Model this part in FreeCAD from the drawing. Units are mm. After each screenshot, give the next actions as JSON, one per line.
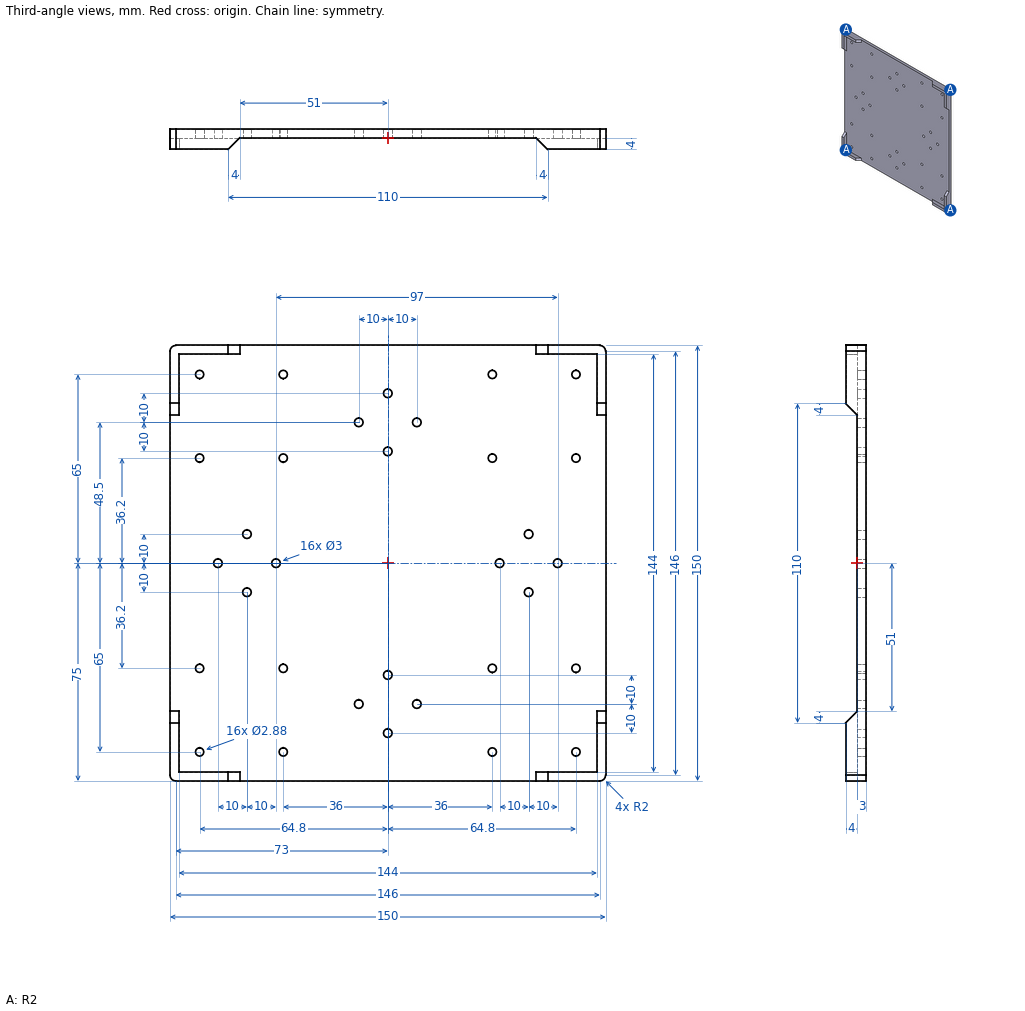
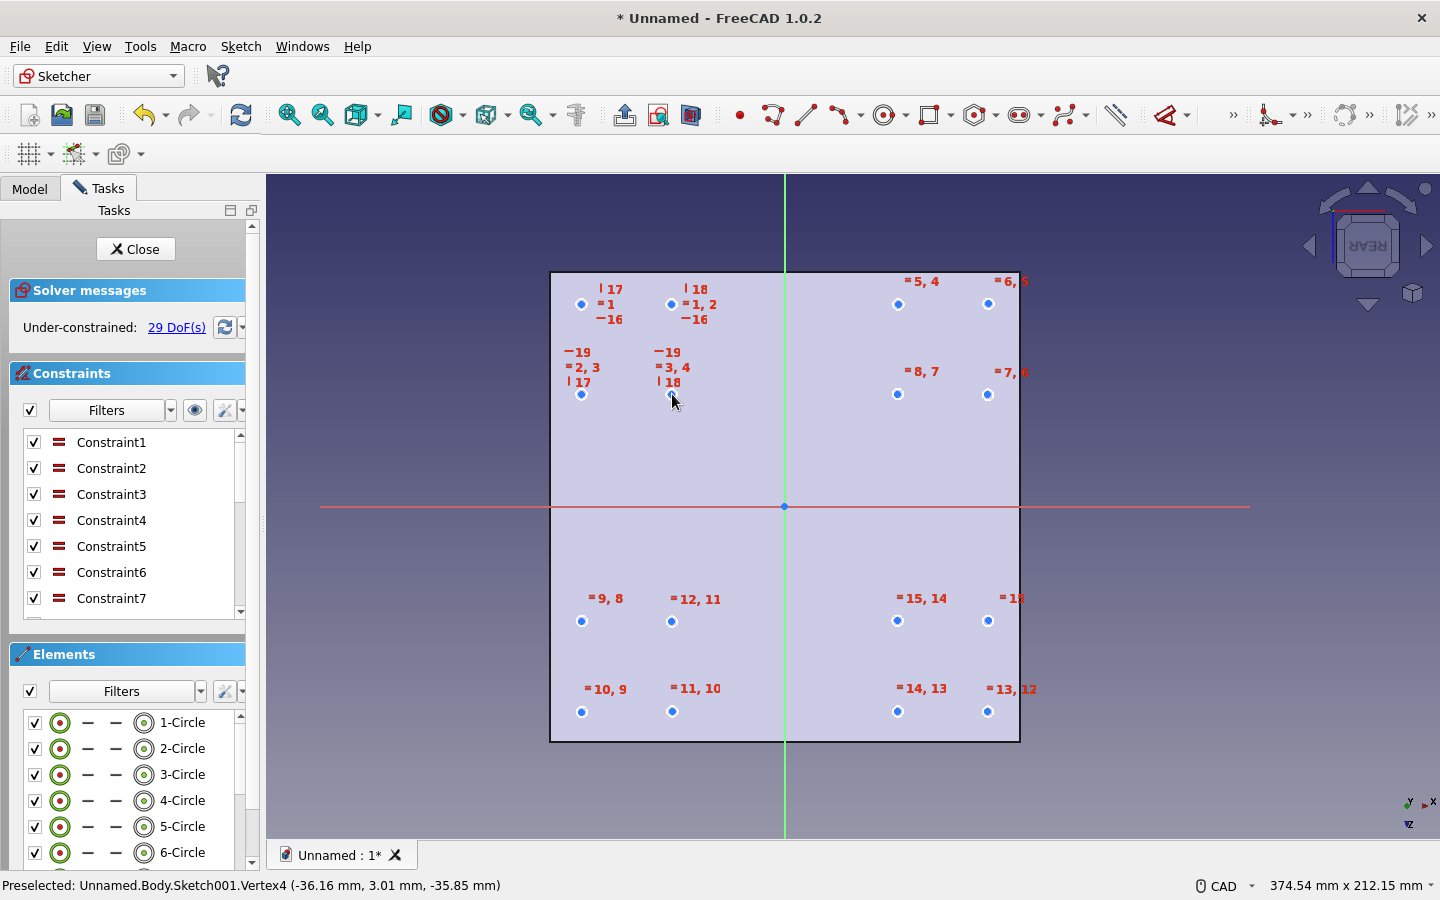
{"action": "left_click", "coordinate": [672, 304]}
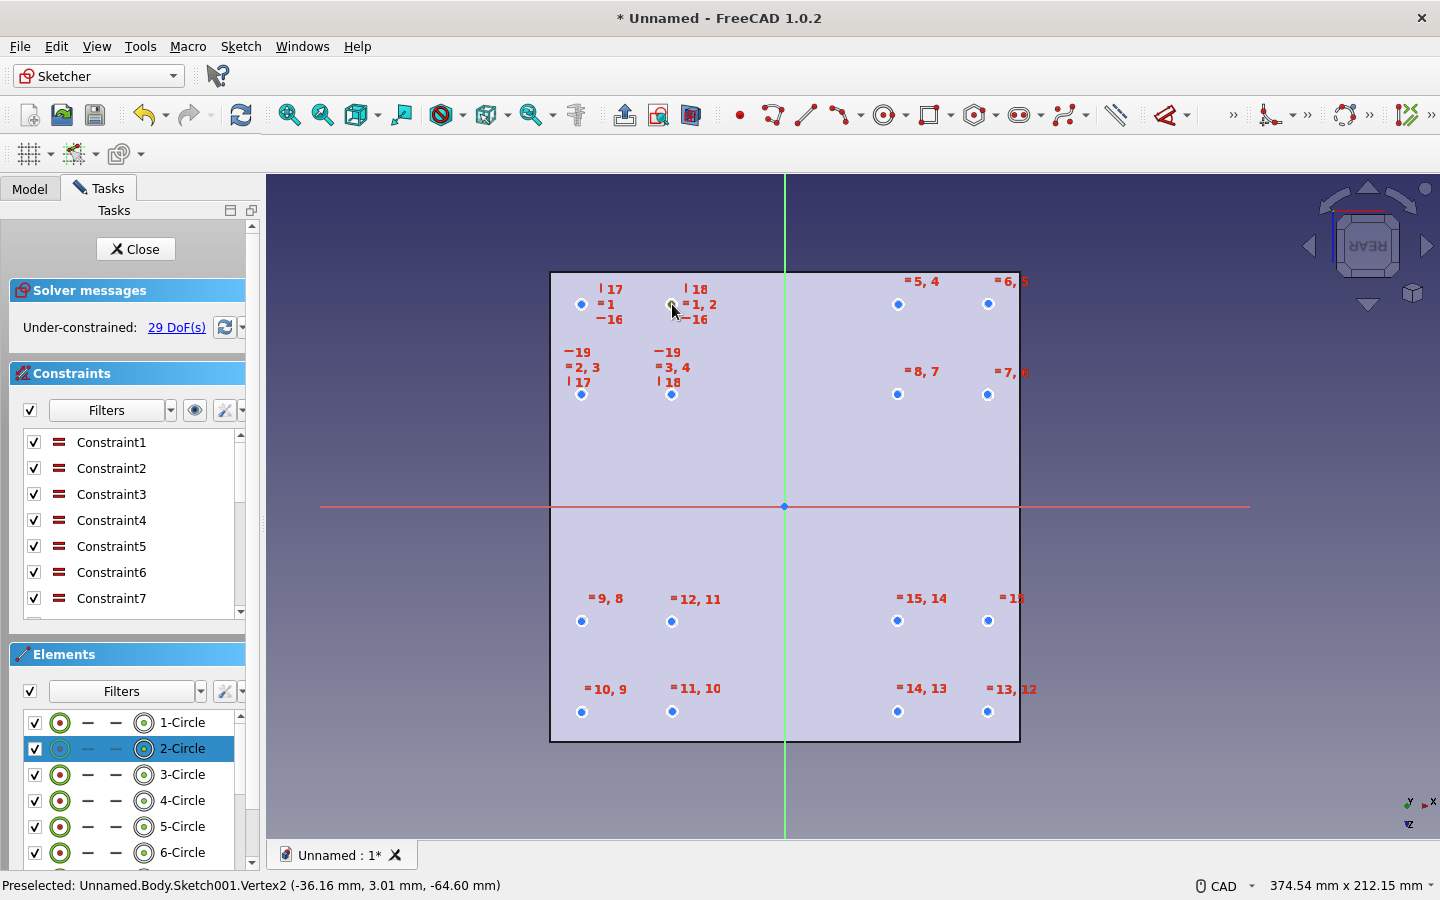
{"action": "left_click", "coordinate": [898, 304]}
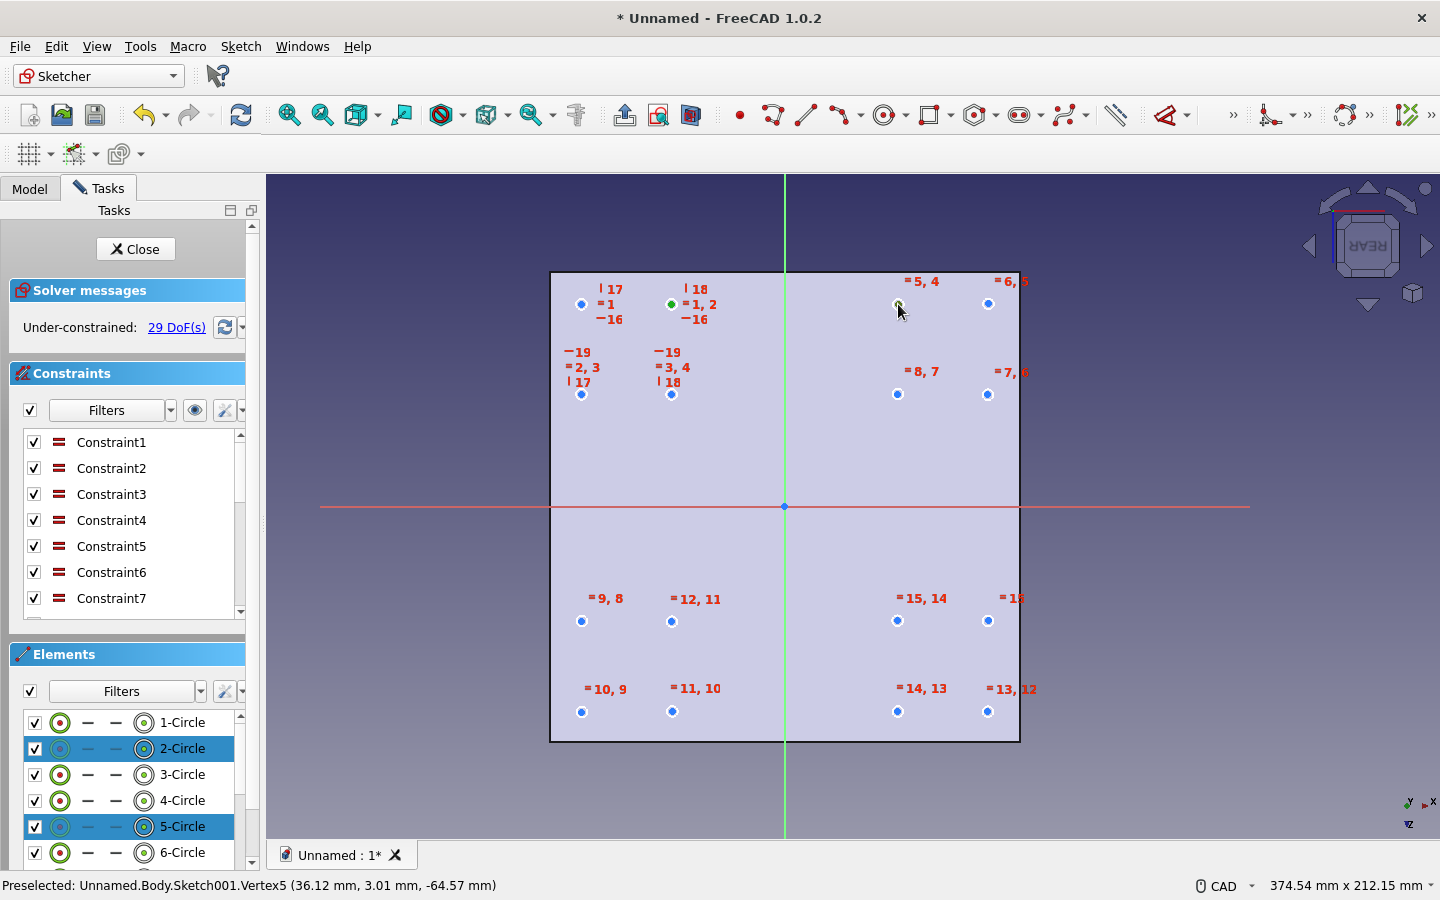
{"action": "key", "text": "h"}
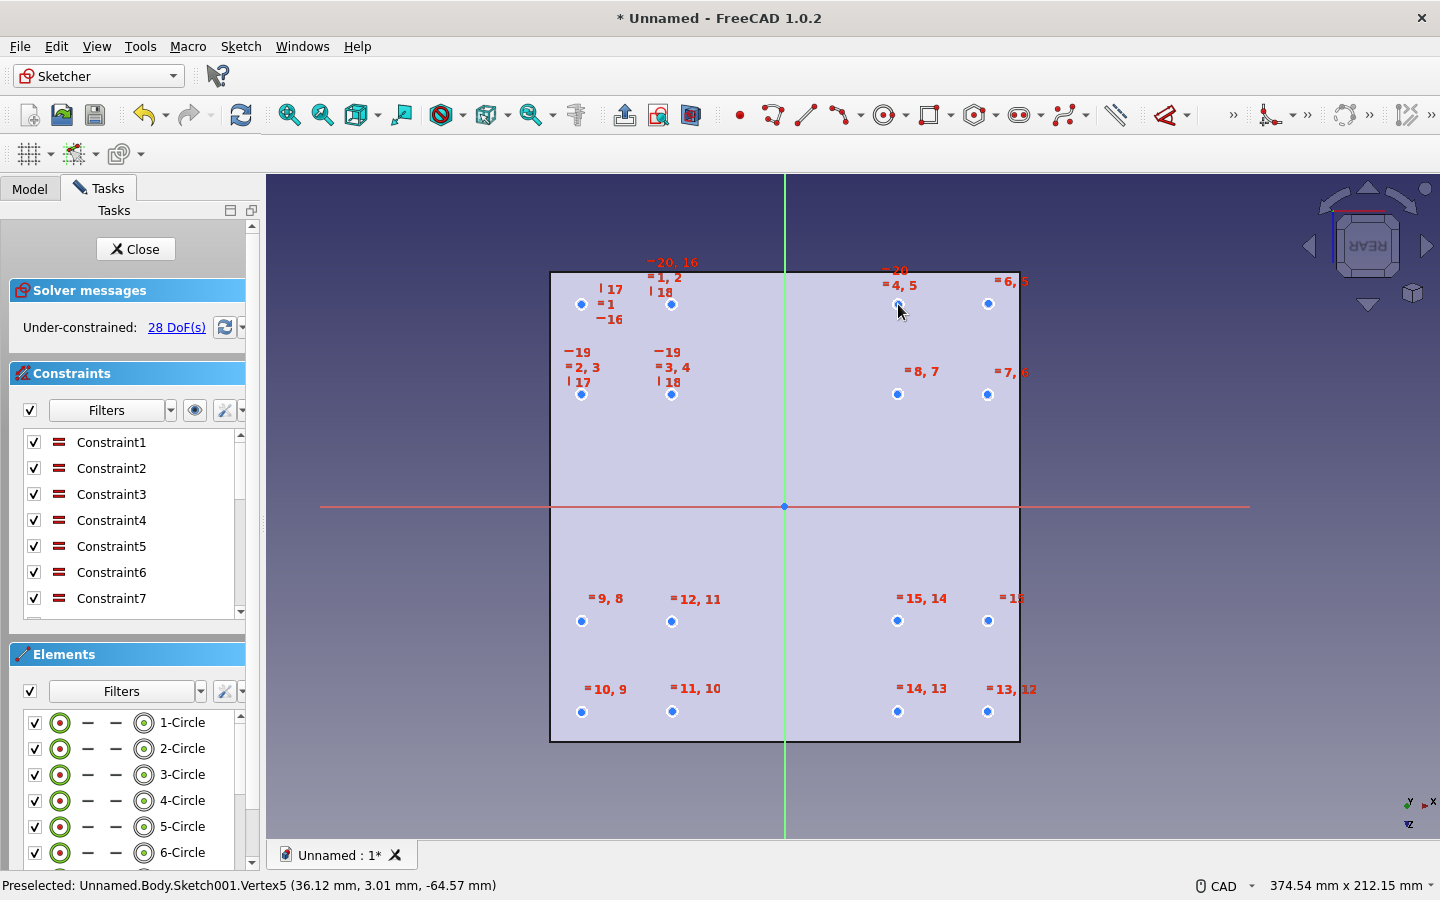
{"action": "left_click", "coordinate": [898, 304]}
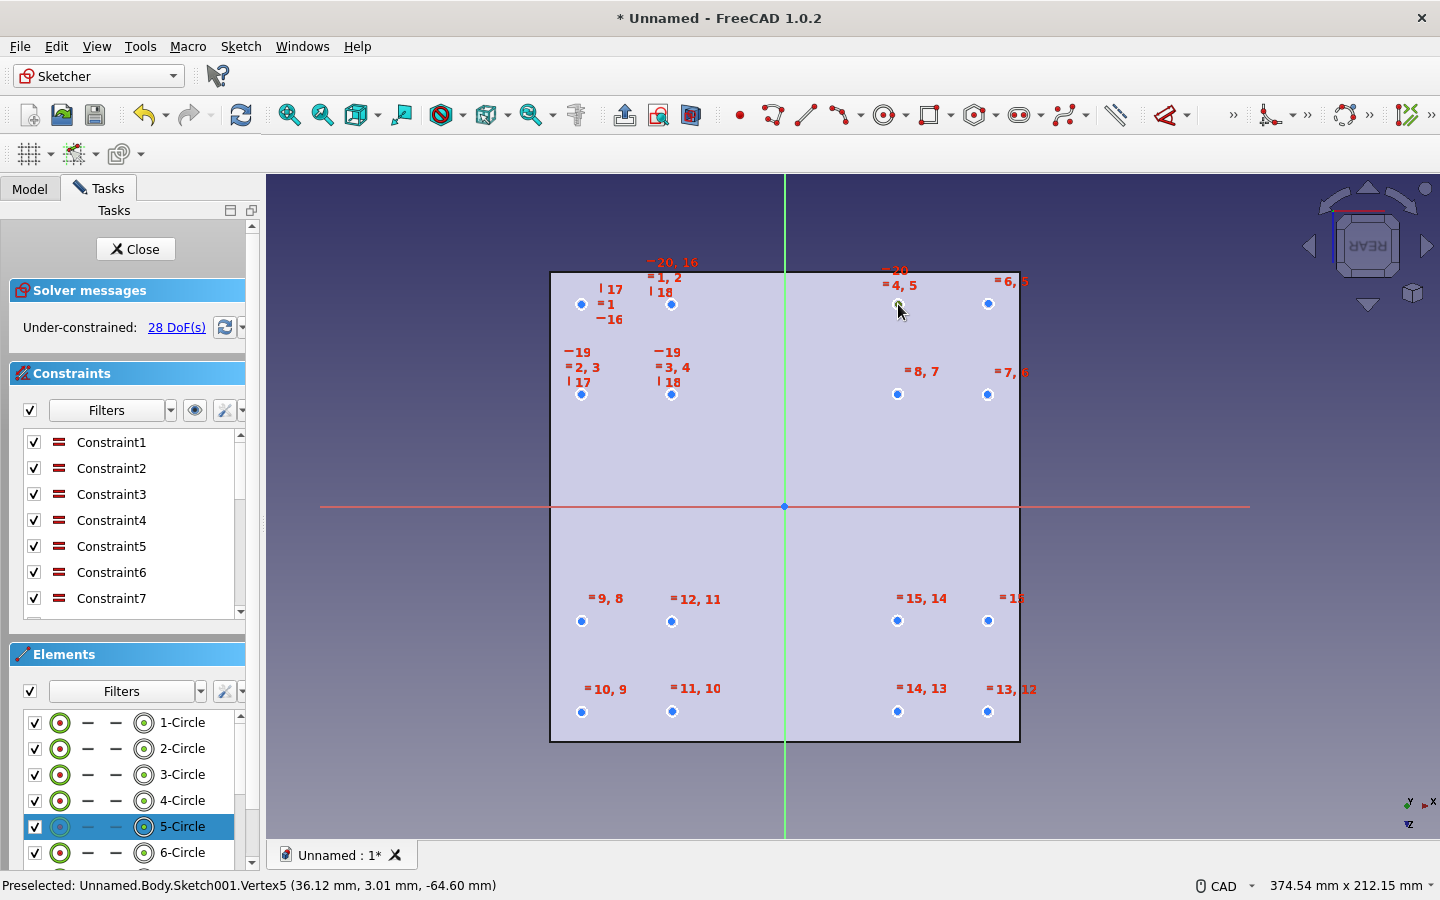
{"action": "left_click", "coordinate": [988, 304]}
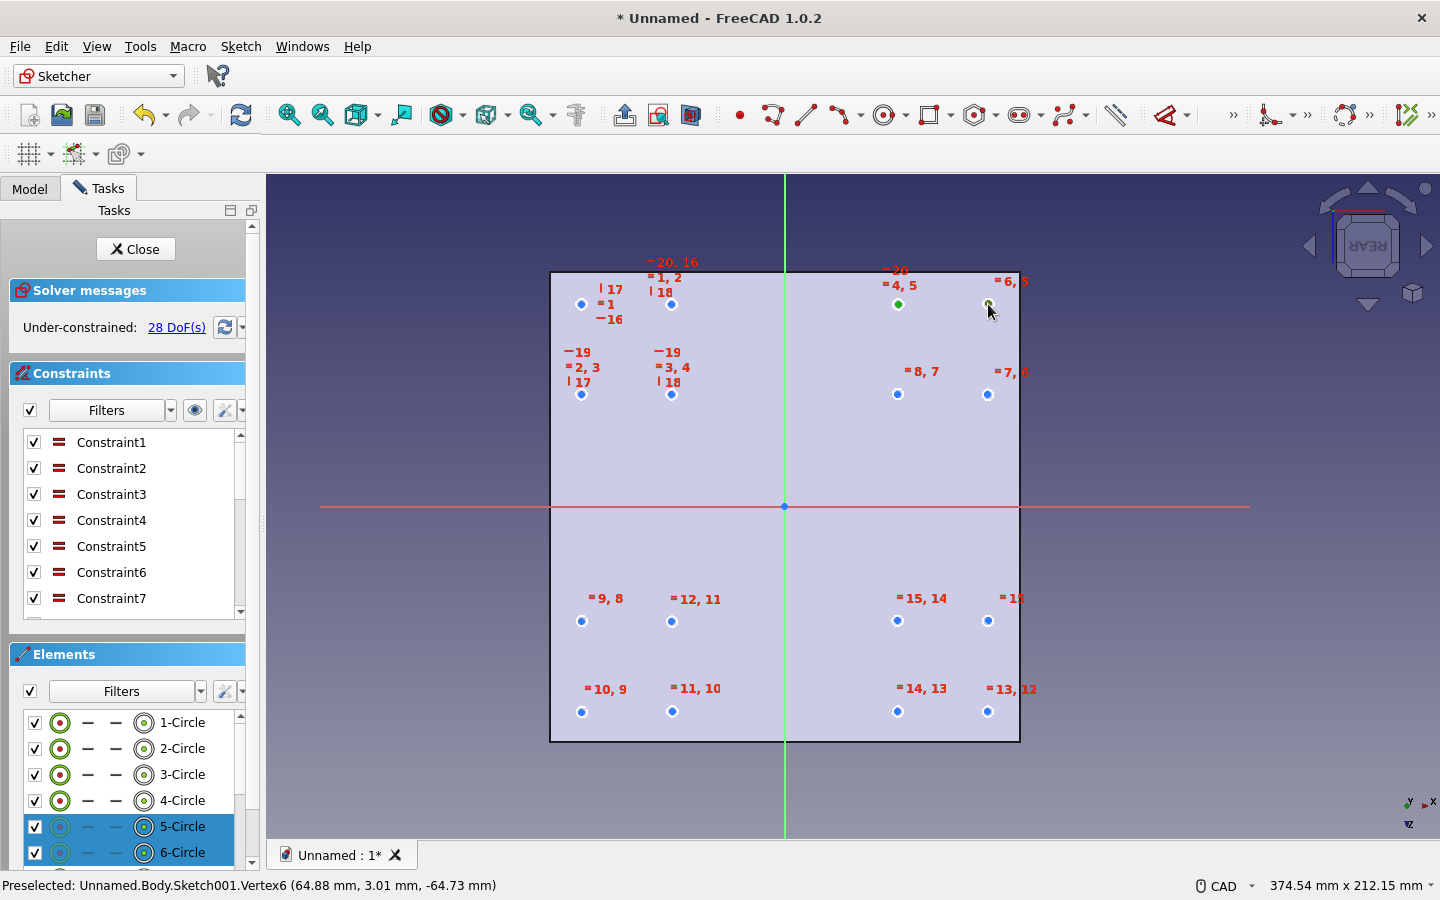
{"action": "key", "text": "h"}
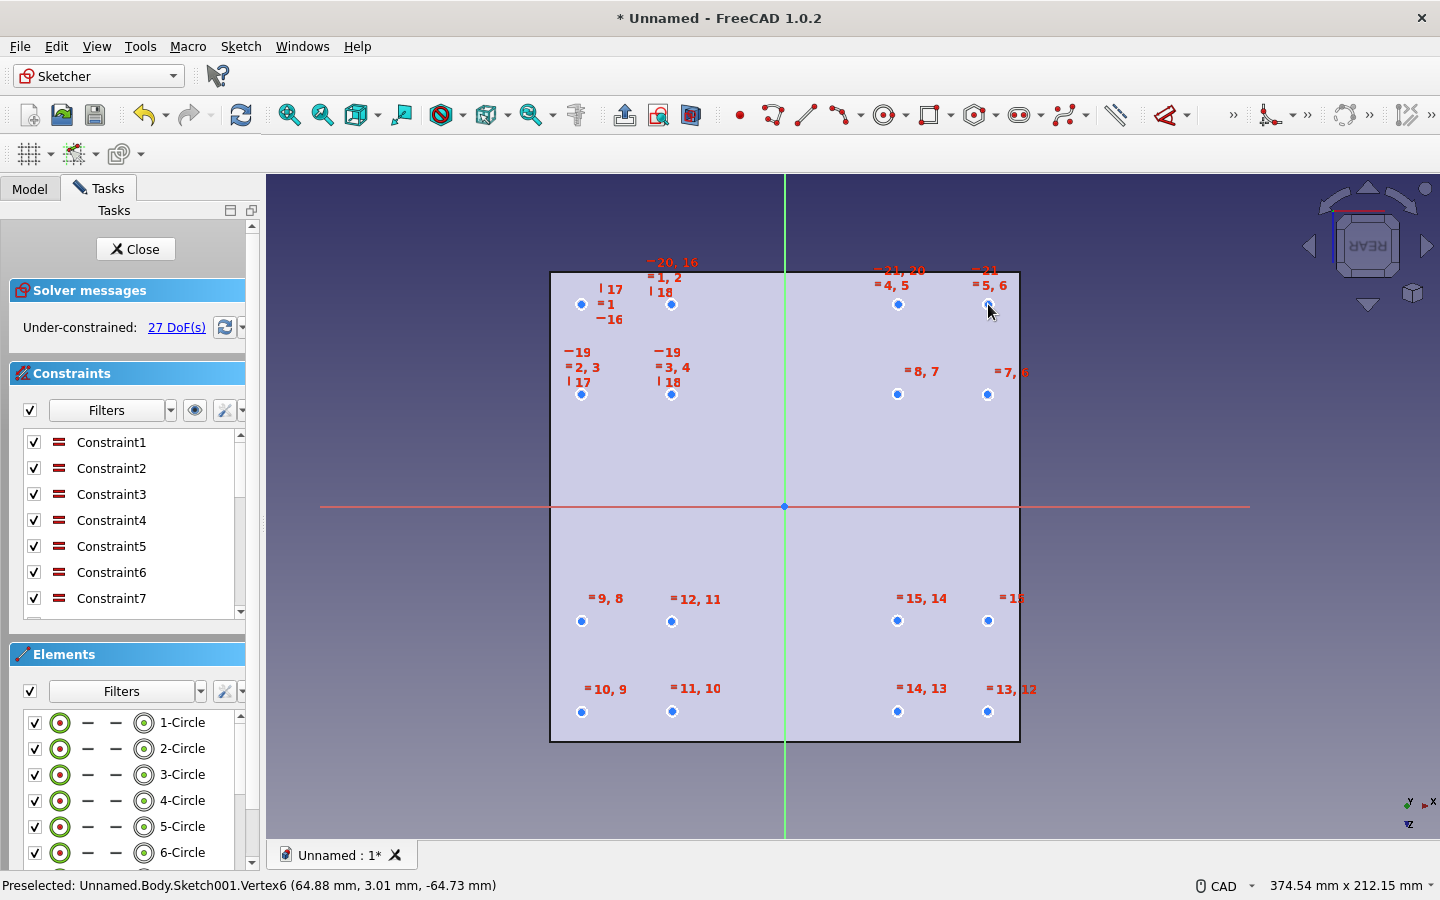
{"action": "left_click", "coordinate": [988, 304]}